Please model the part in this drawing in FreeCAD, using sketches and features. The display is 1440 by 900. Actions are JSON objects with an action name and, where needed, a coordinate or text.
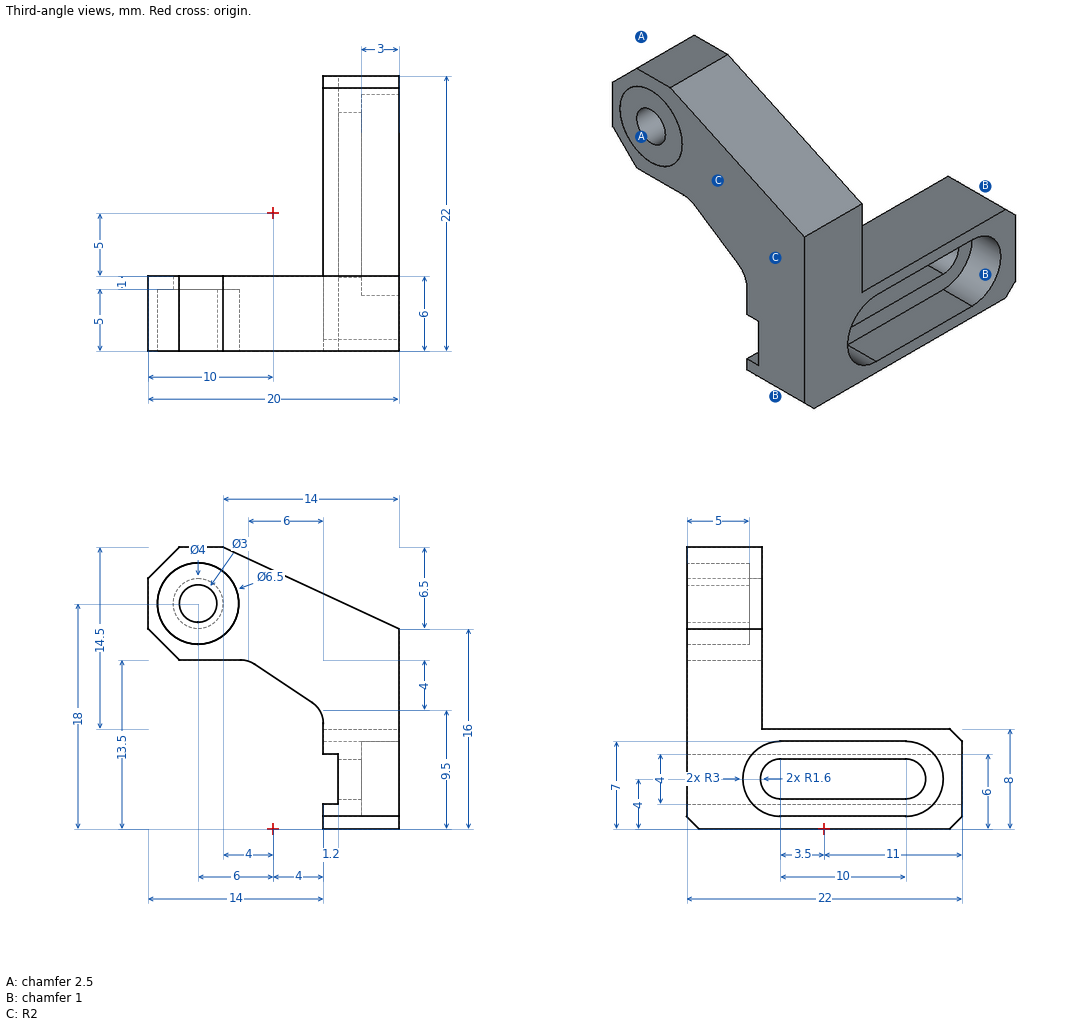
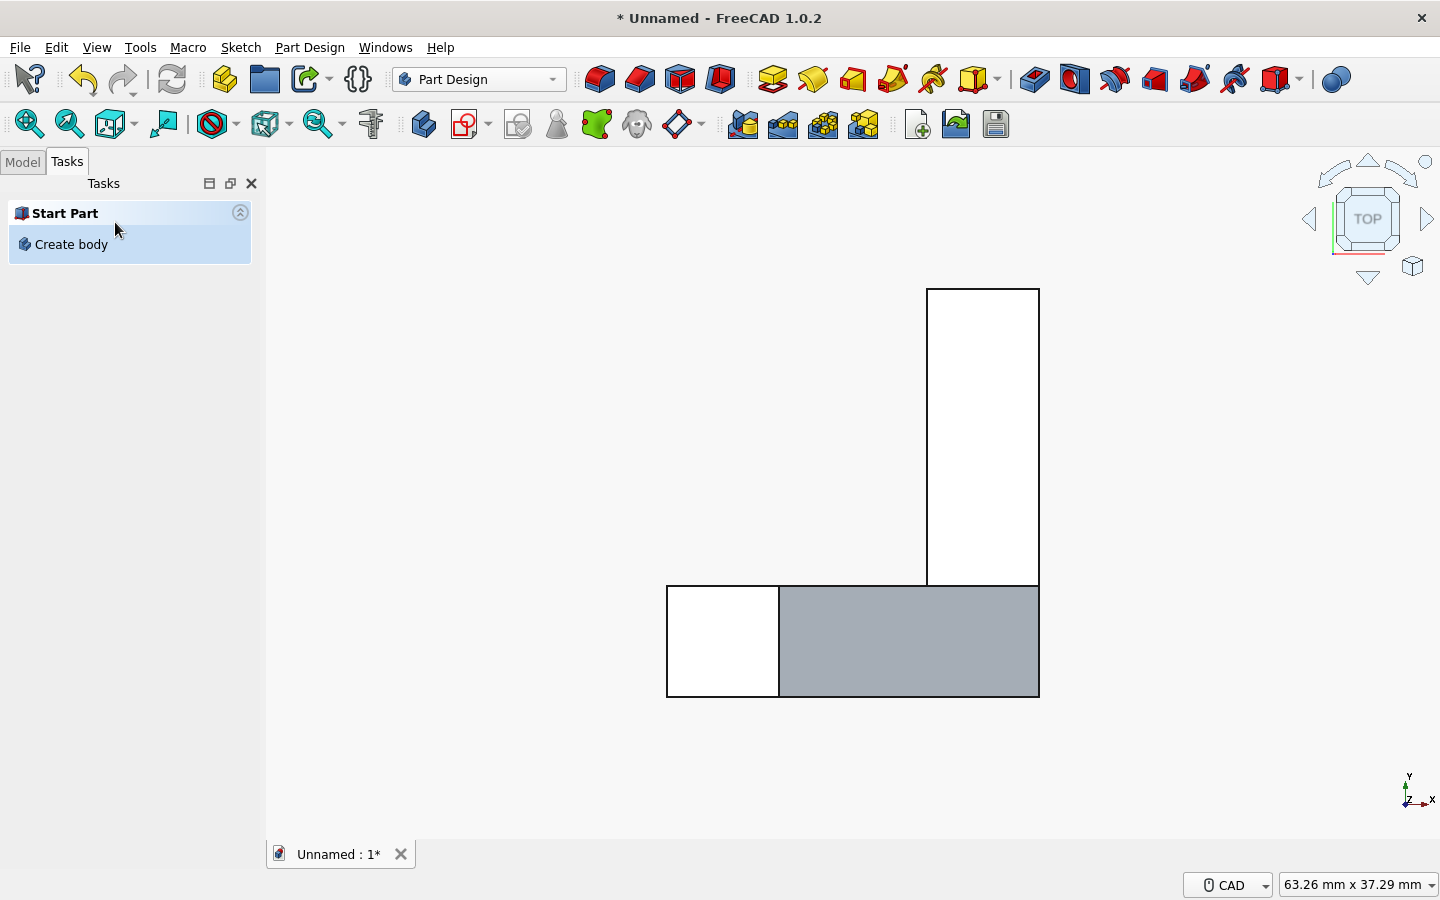
{"action": "left_click", "coordinate": [667, 640]}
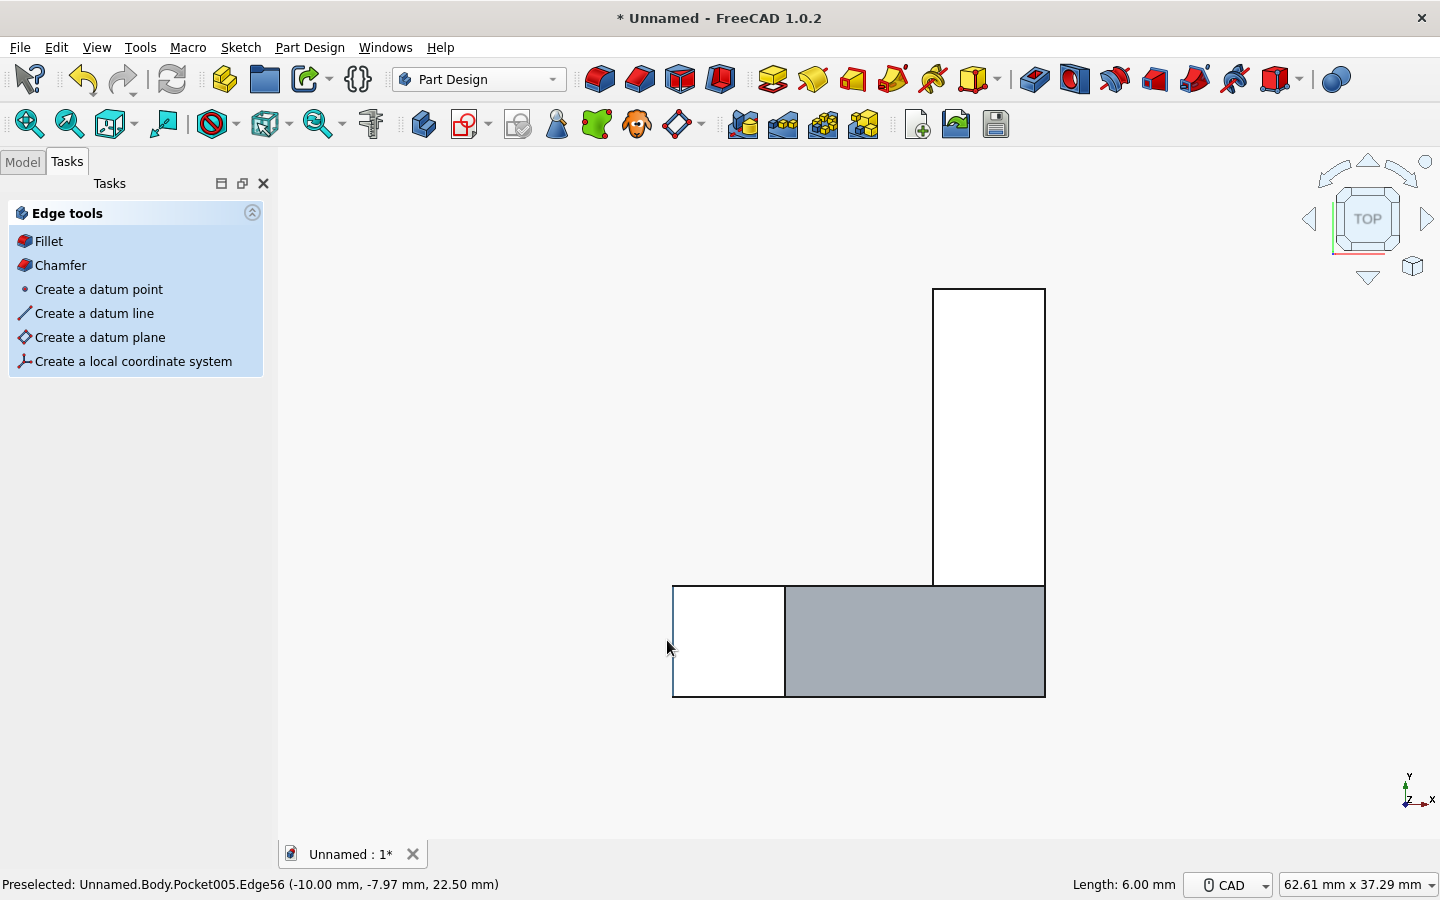
{"action": "key", "text": "0"}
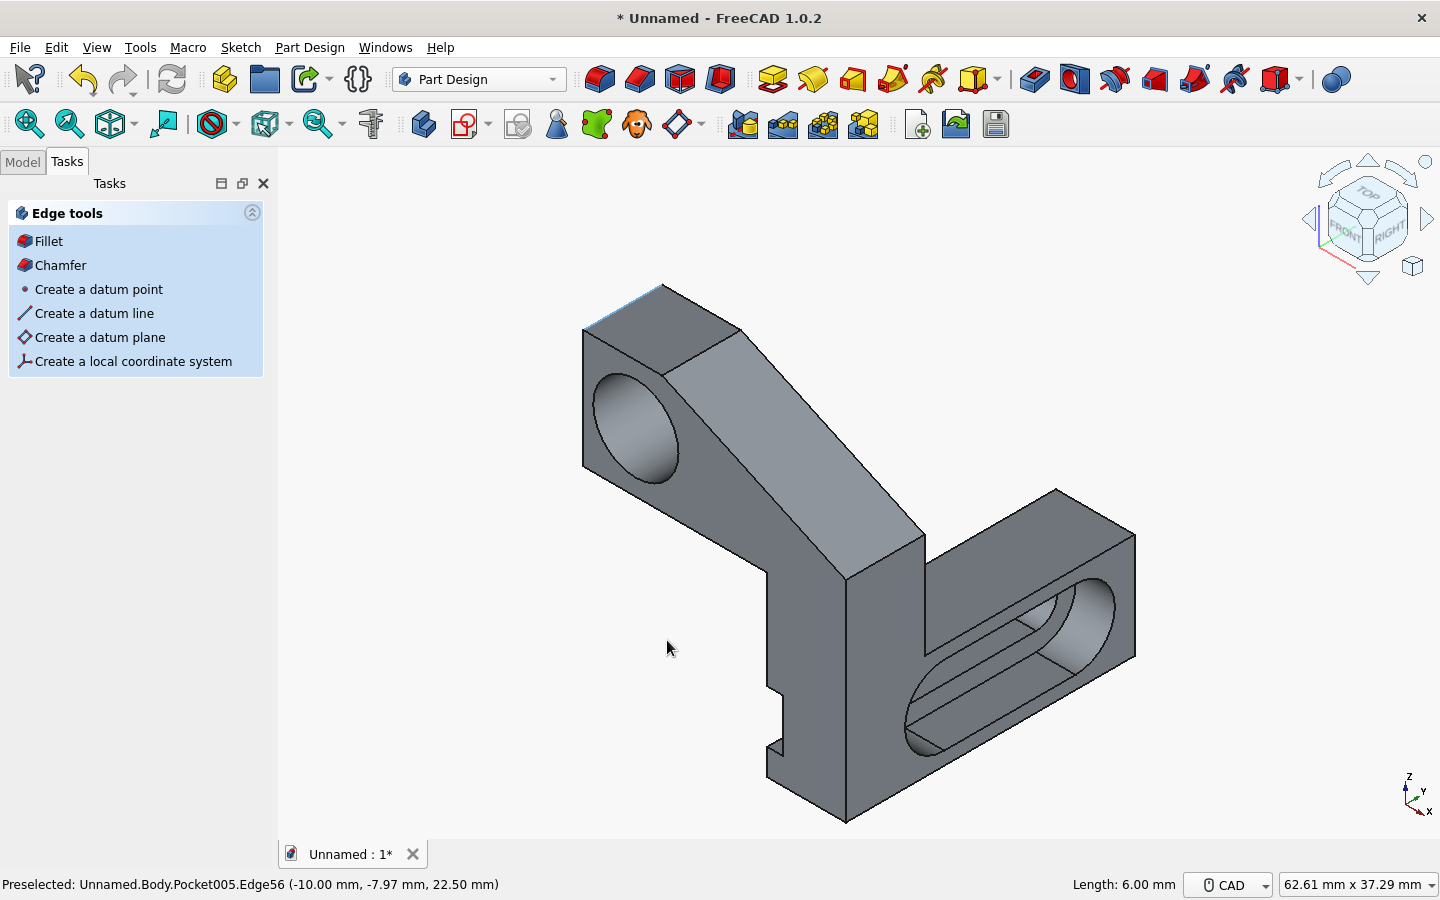
{"action": "key", "text": "1"}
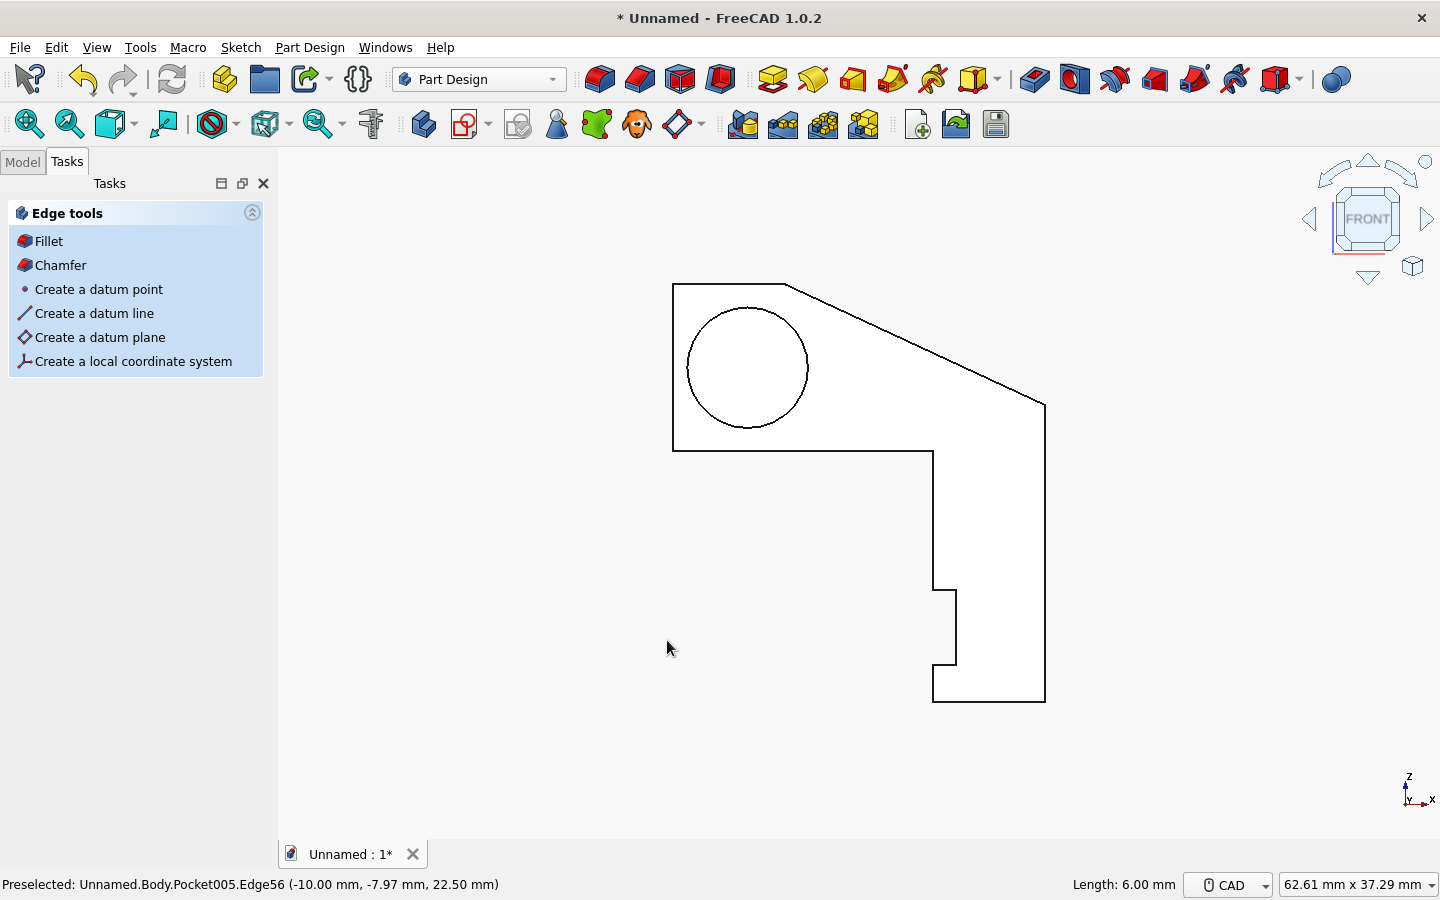
{"action": "key", "text": "3"}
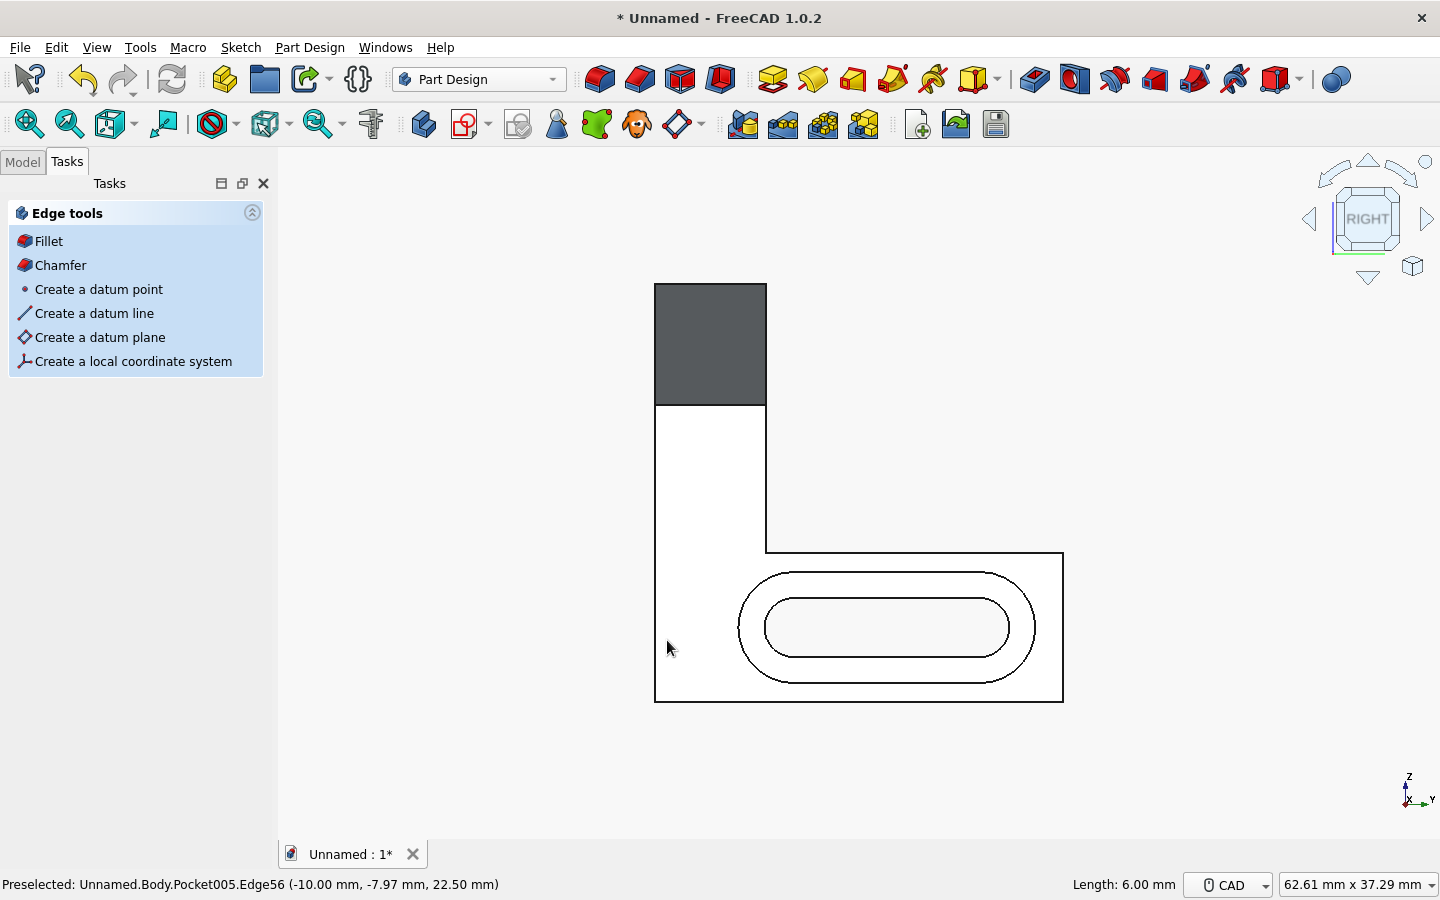
{"action": "key", "text": "5"}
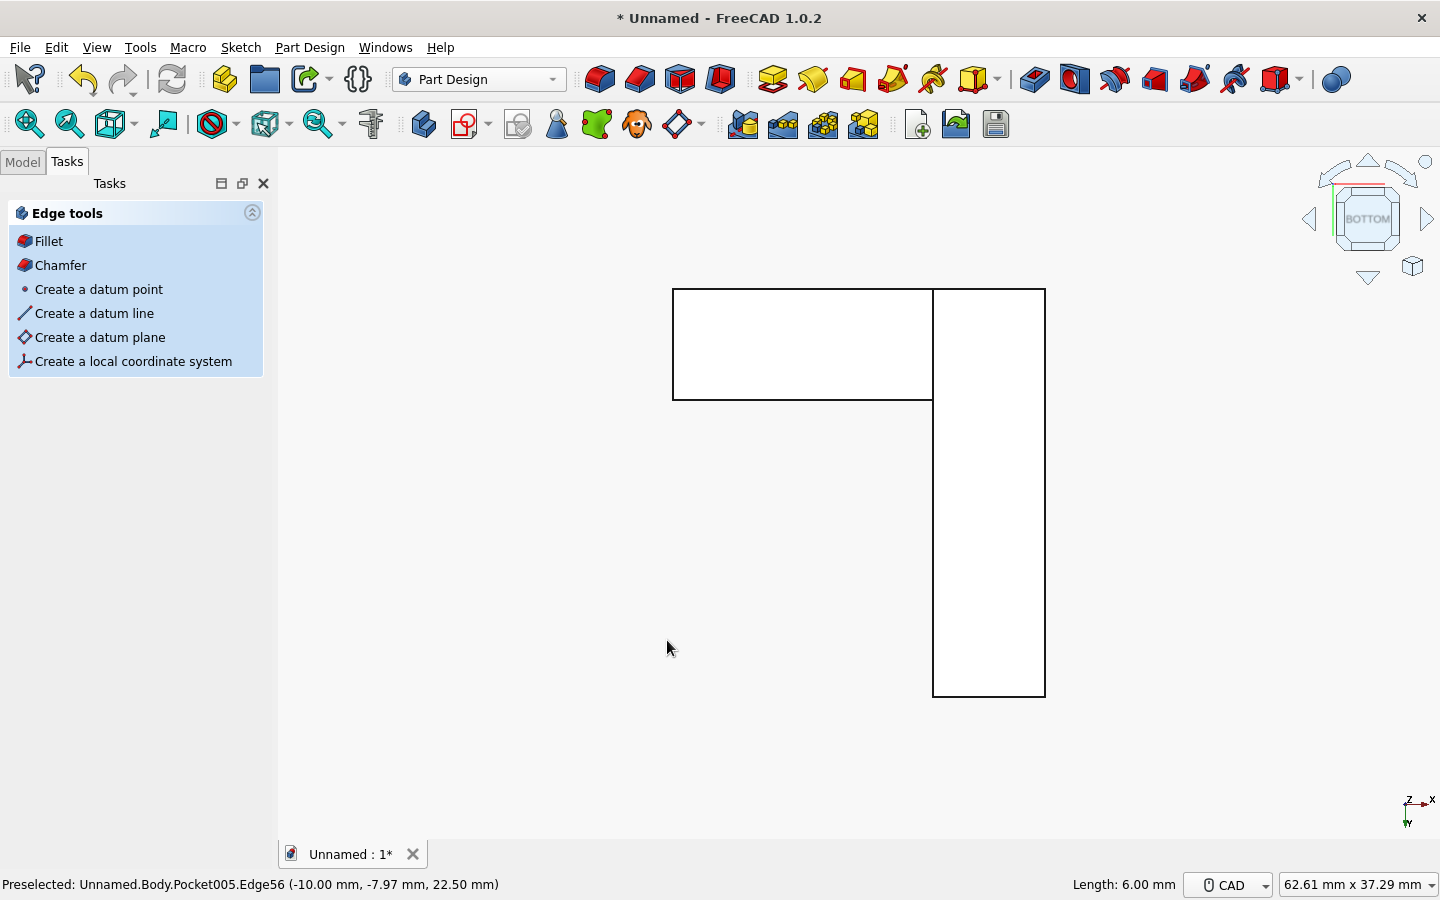
{"action": "left_click", "coordinate": [673, 344], "text": "ctrl"}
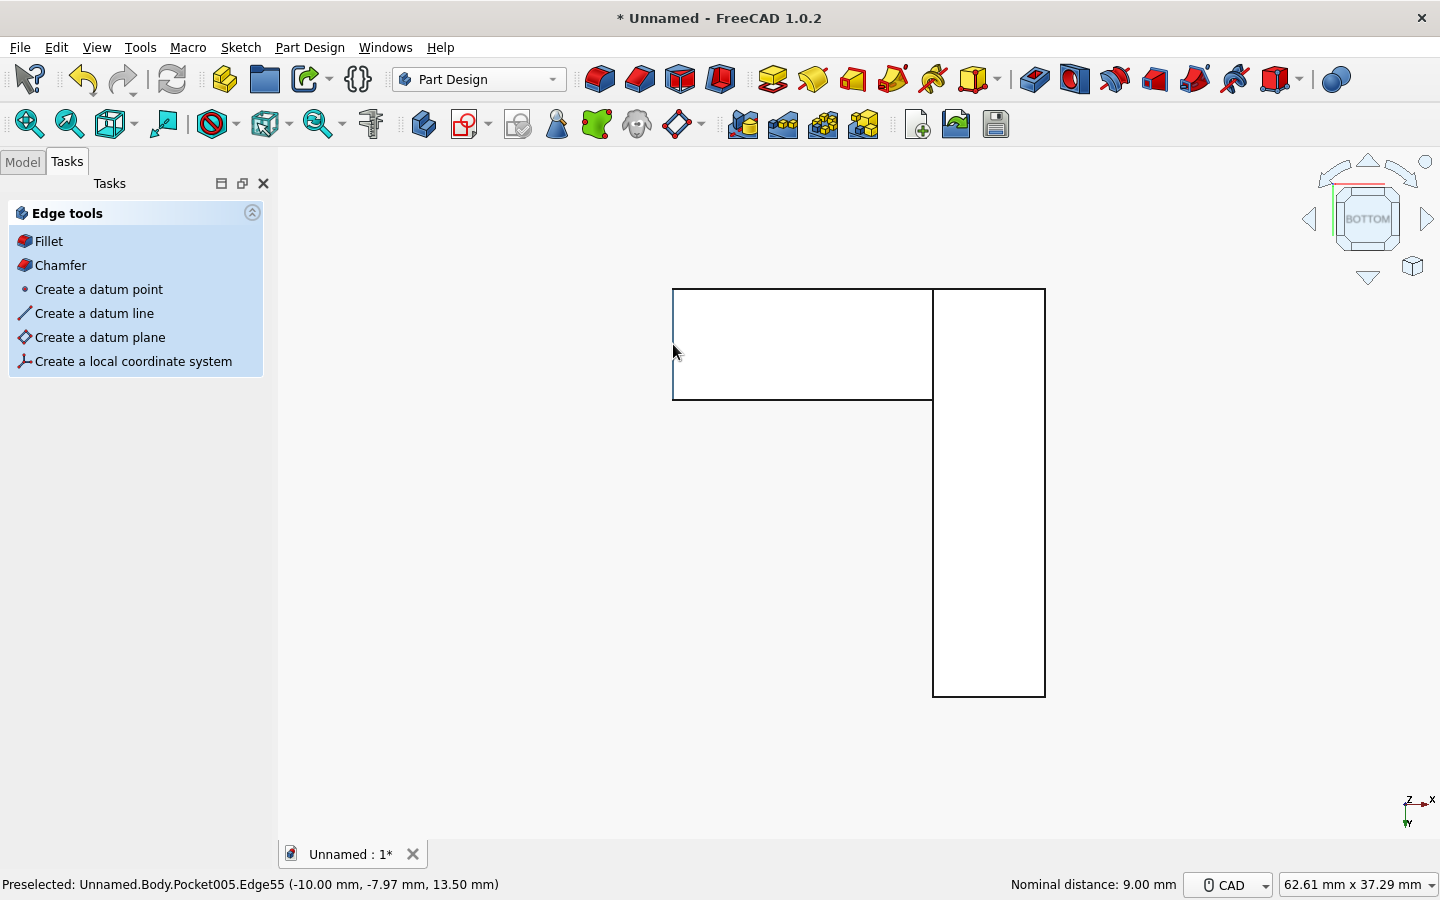
{"action": "left_click", "coordinate": [640, 80]}